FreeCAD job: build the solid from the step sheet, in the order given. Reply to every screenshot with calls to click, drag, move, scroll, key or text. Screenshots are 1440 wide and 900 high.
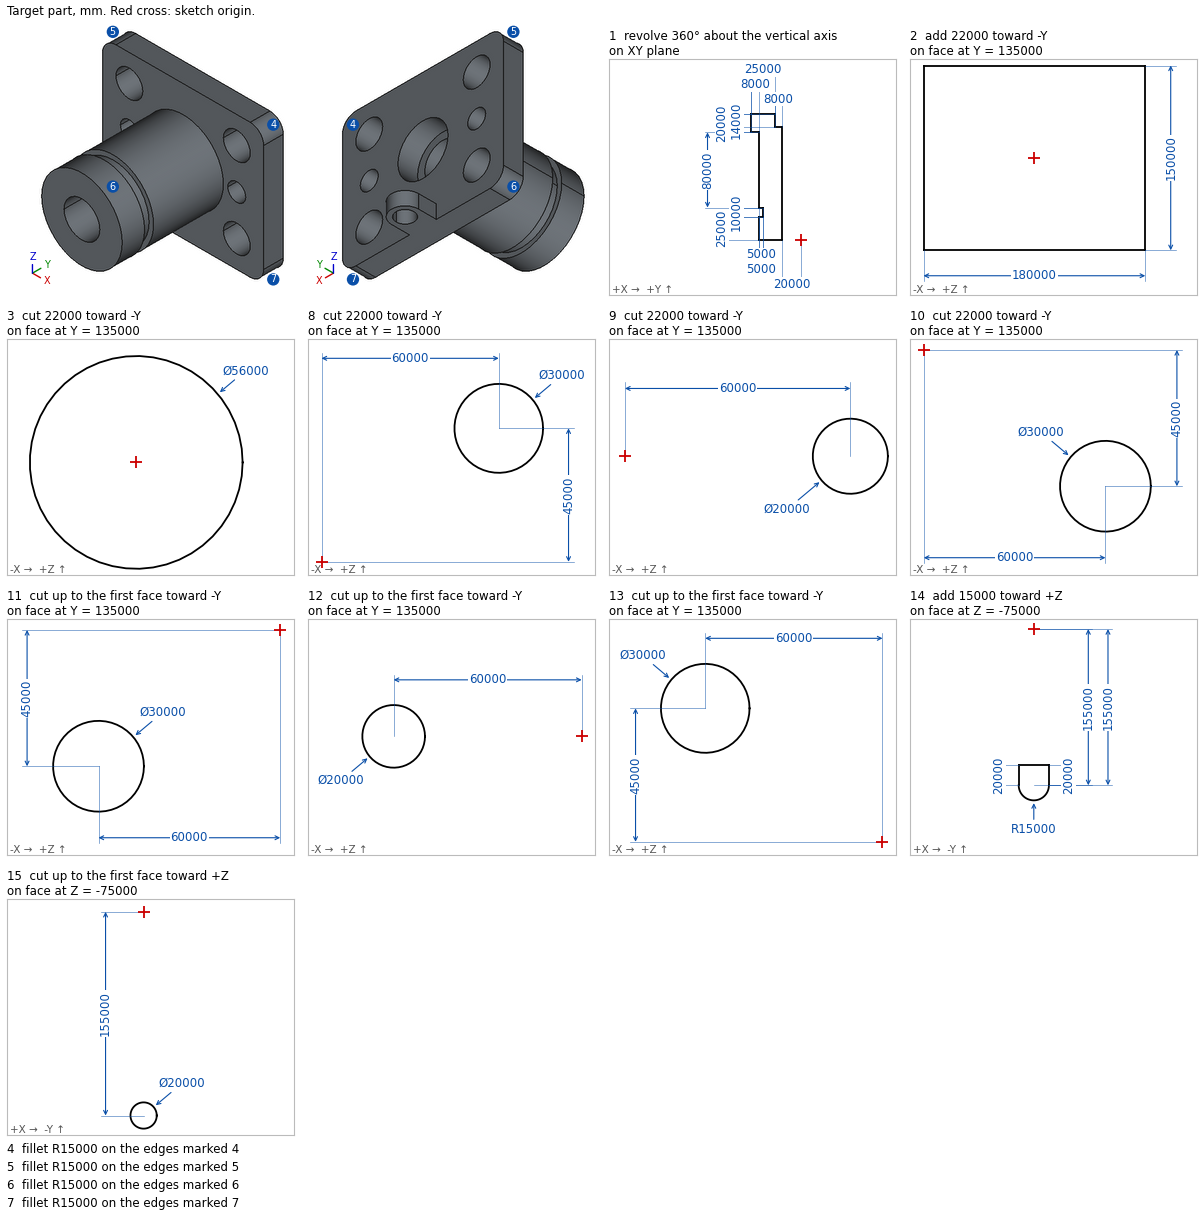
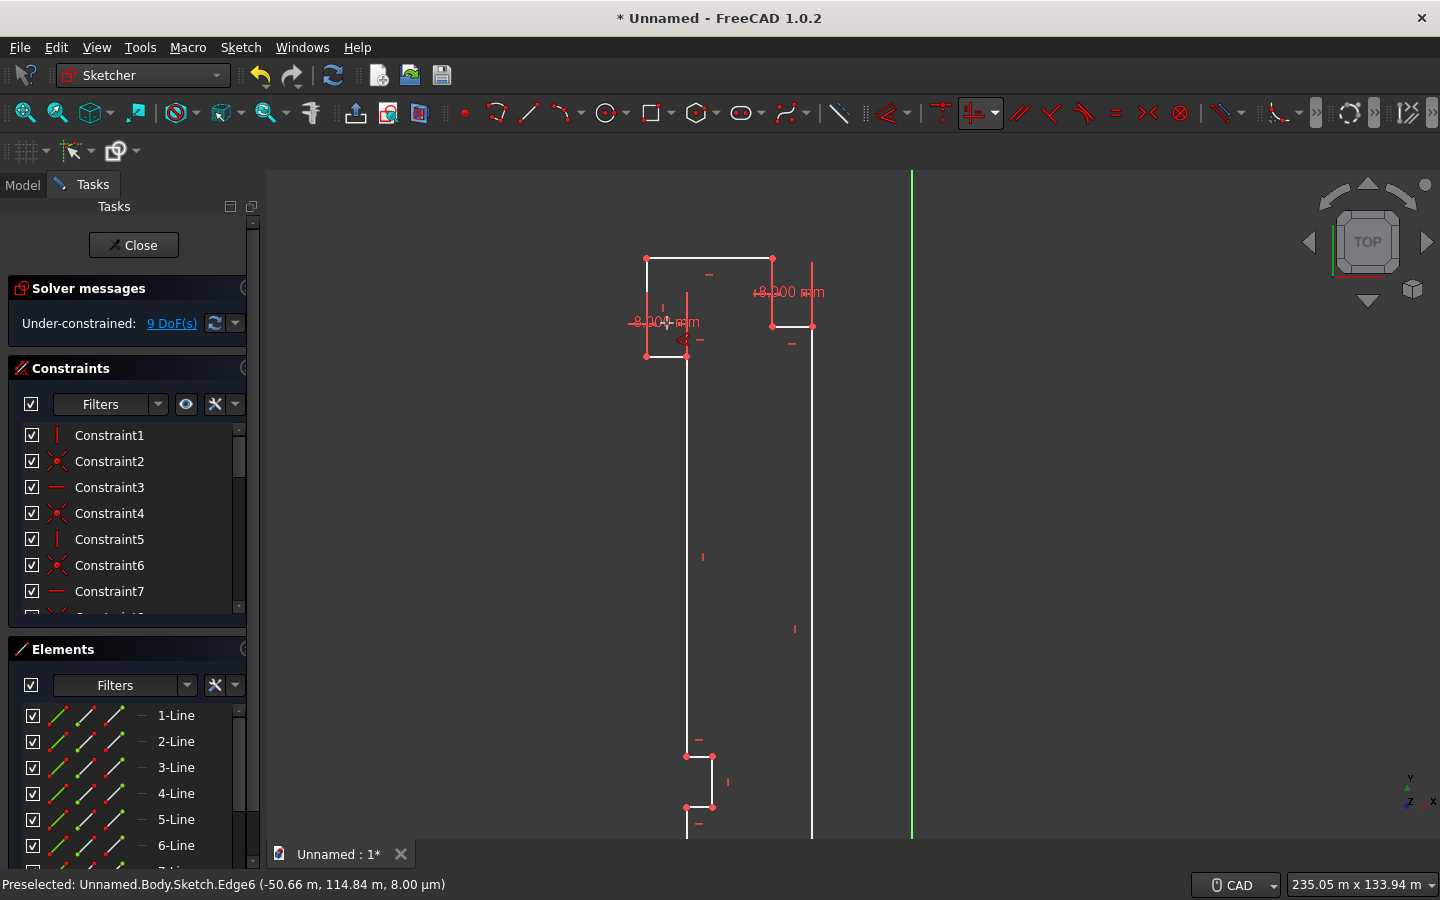
scroll(697, 757, up, 3)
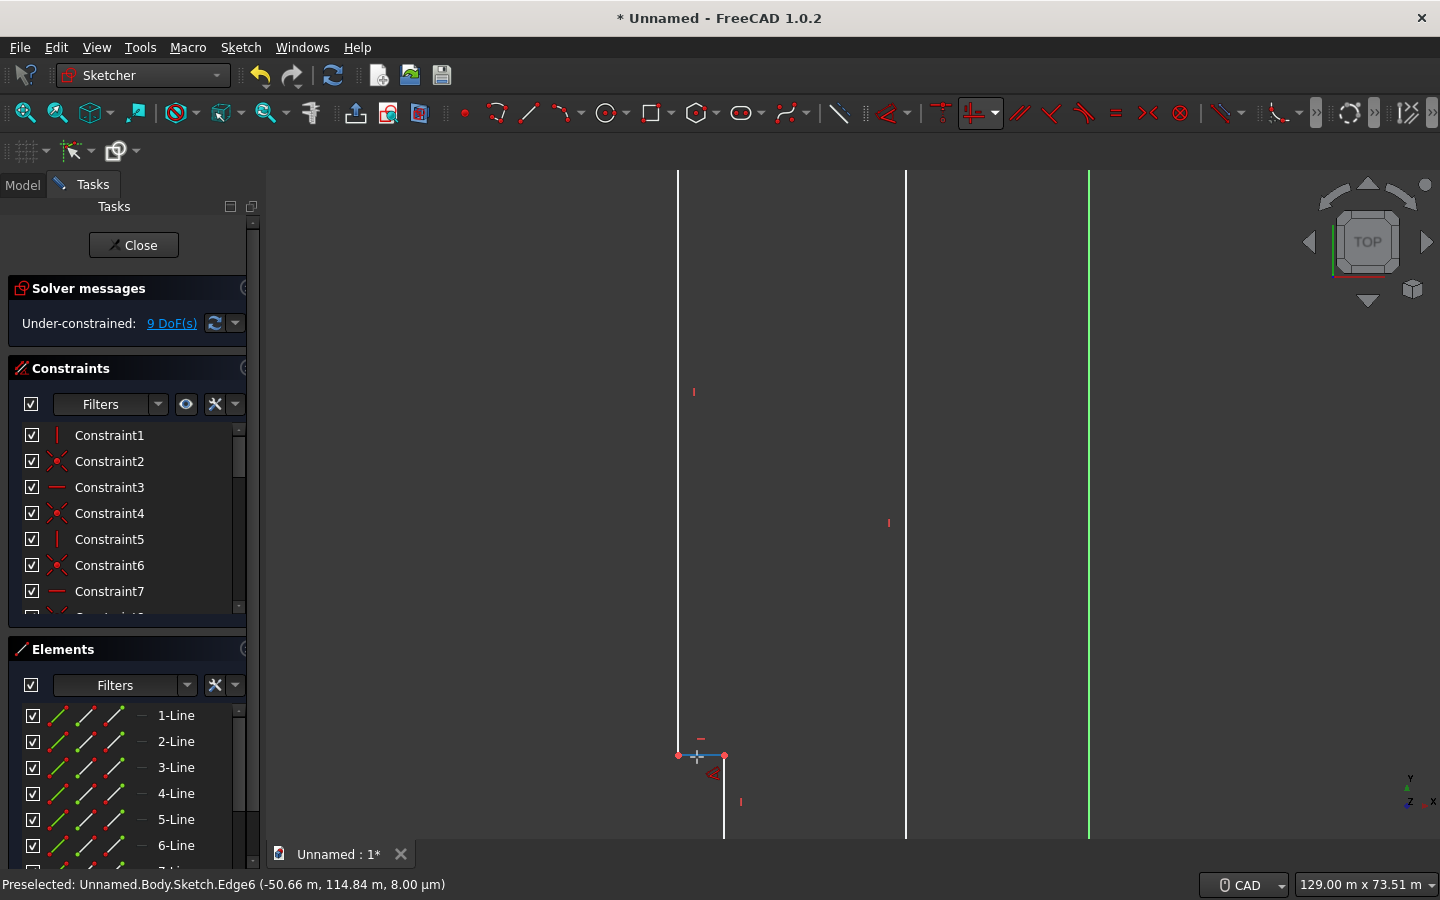
click(697, 755)
click(701, 789)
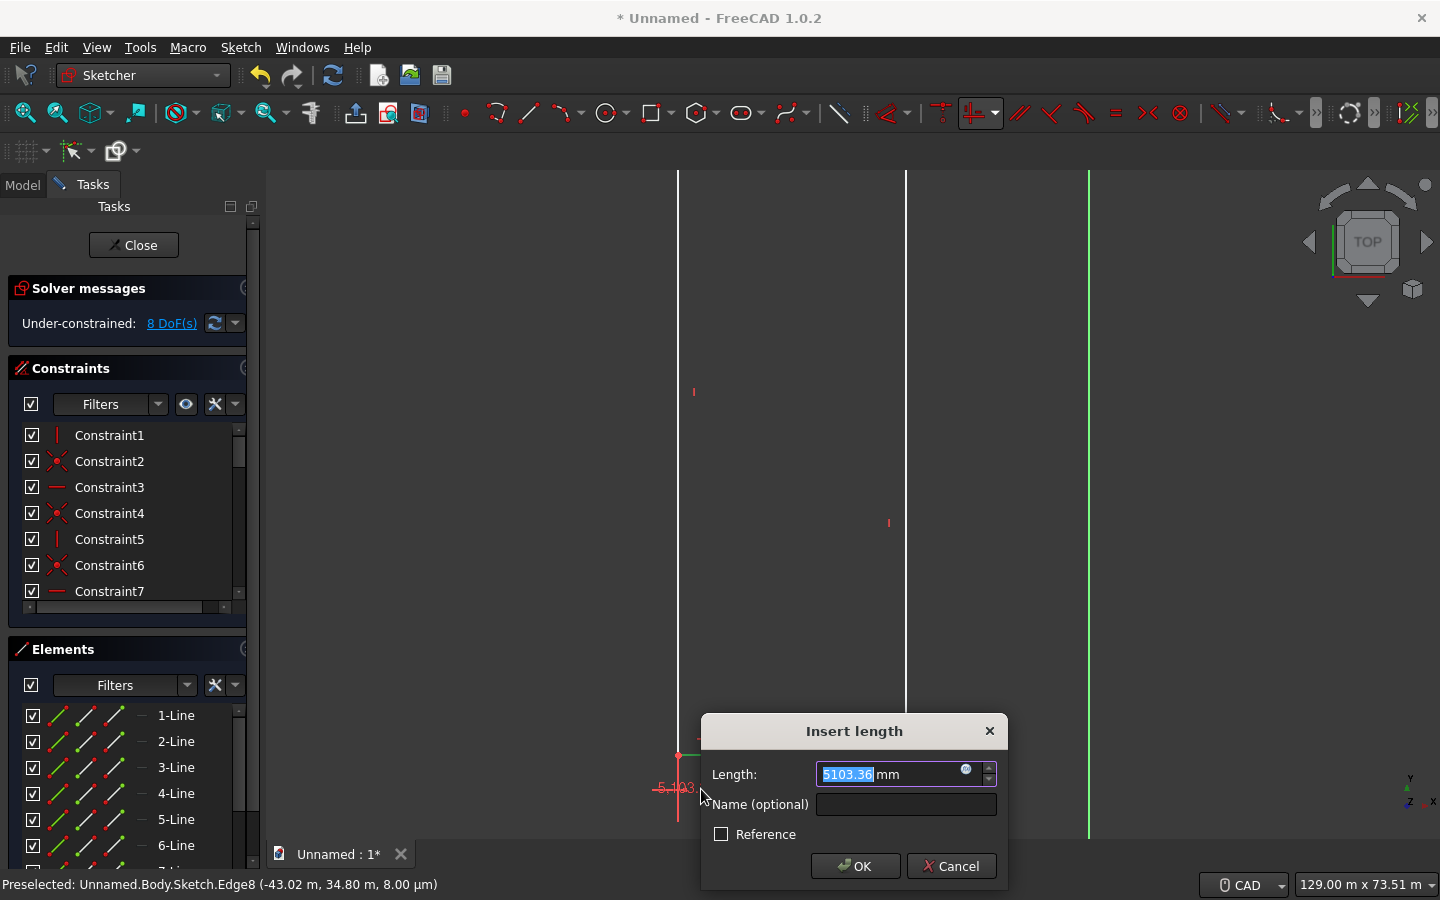
text(5000)
key(Return)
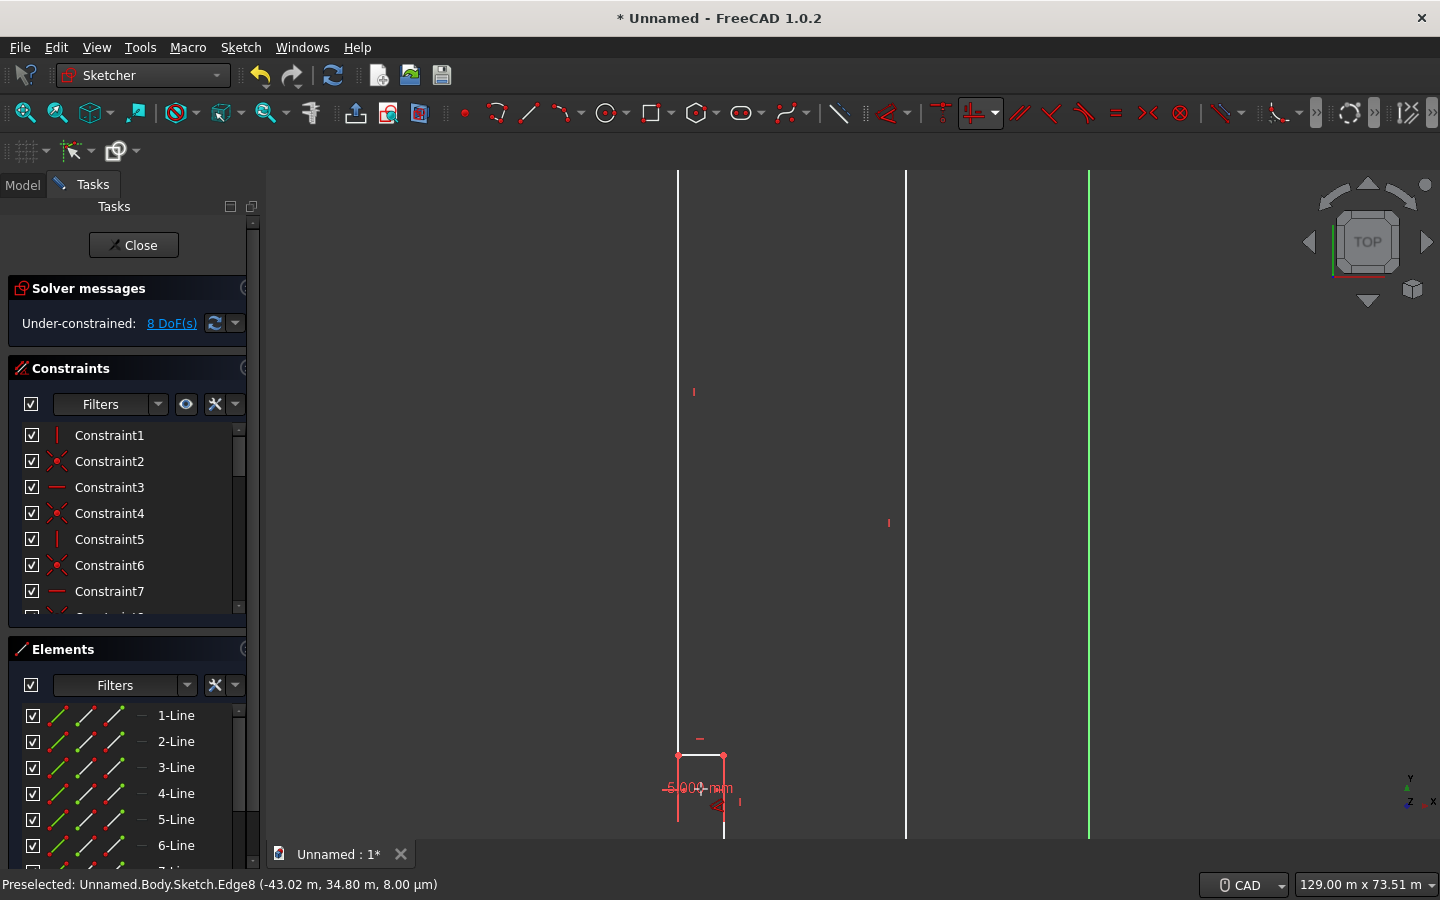
scroll(748, 532, down, 5)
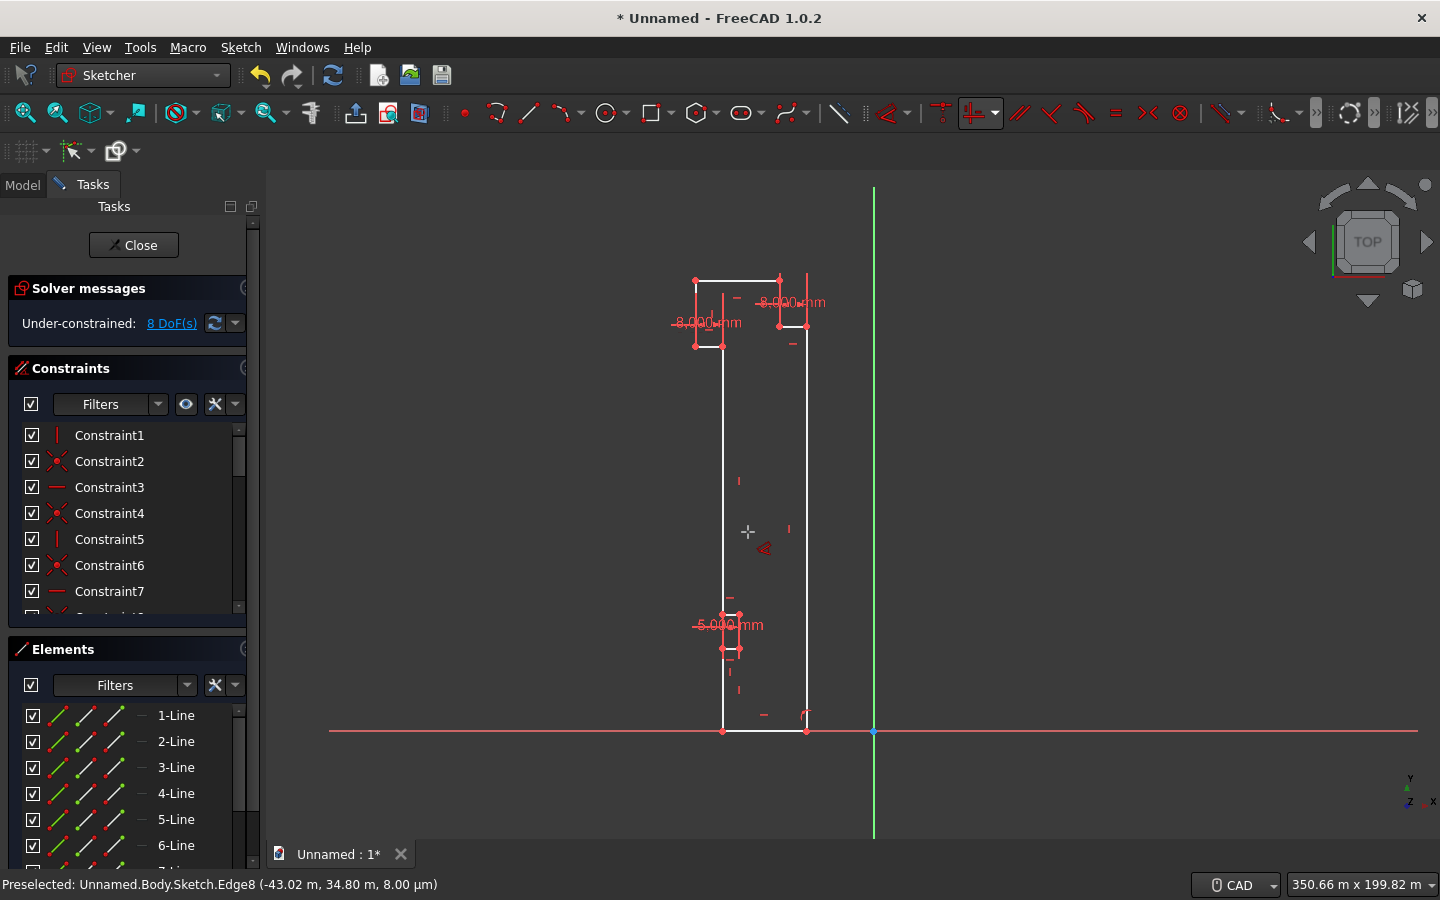
scroll(734, 649, up, 6)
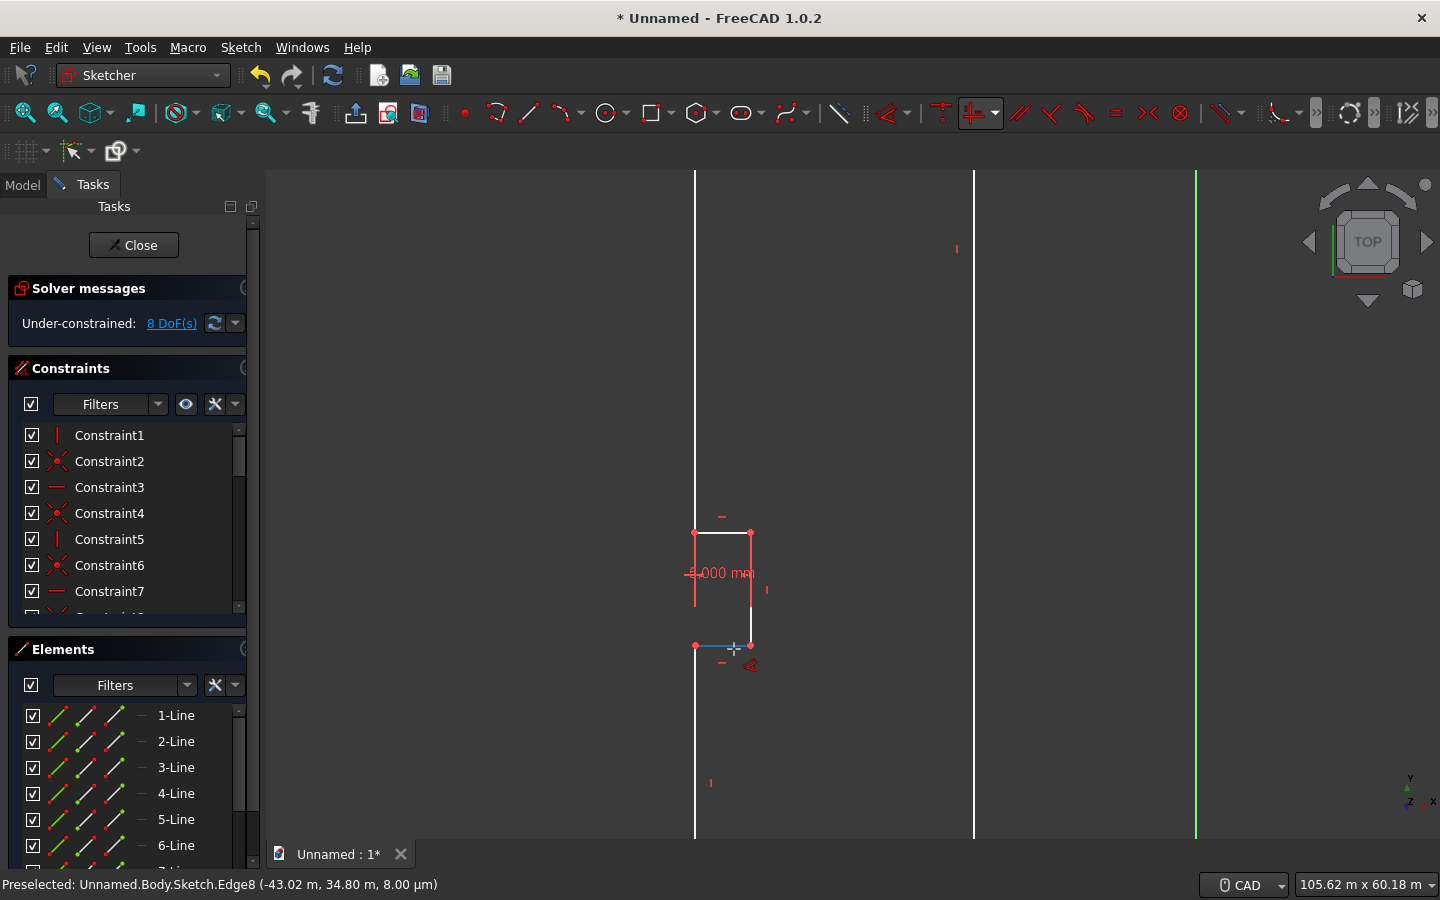
click(734, 646)
click(723, 680)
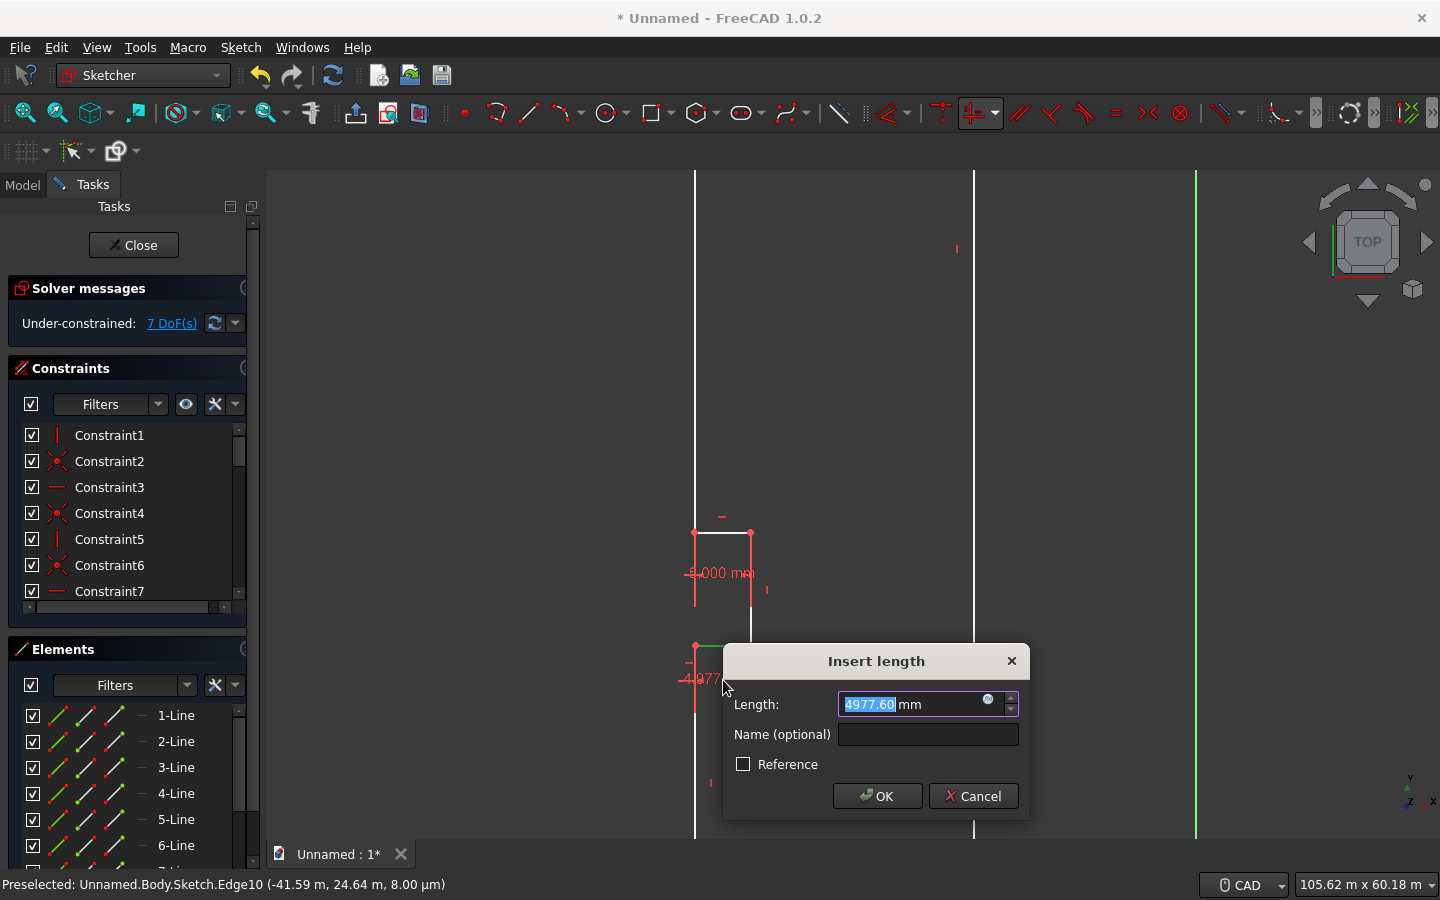
text(5000)
key(Return)